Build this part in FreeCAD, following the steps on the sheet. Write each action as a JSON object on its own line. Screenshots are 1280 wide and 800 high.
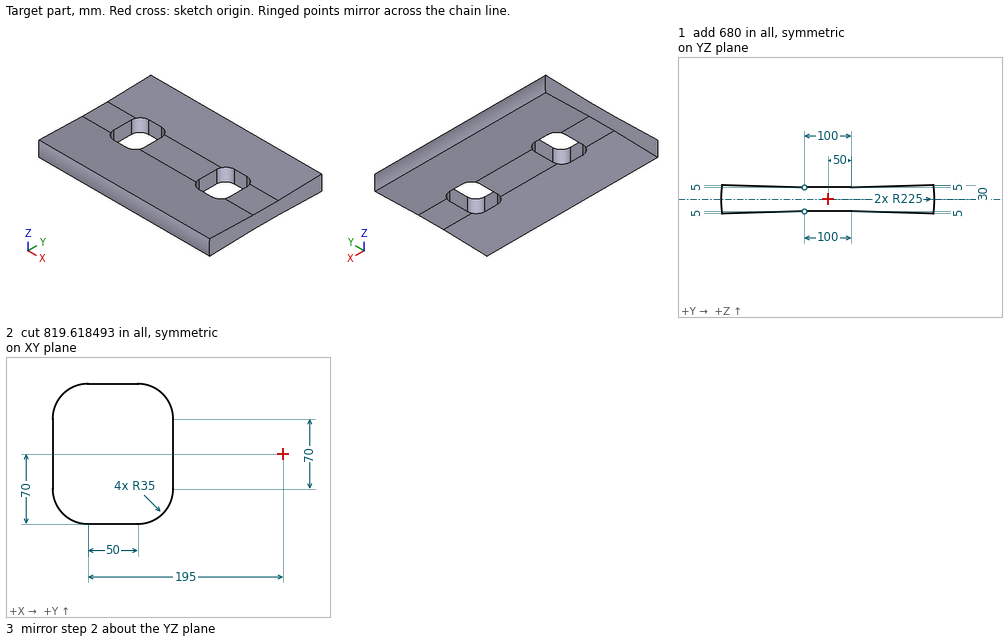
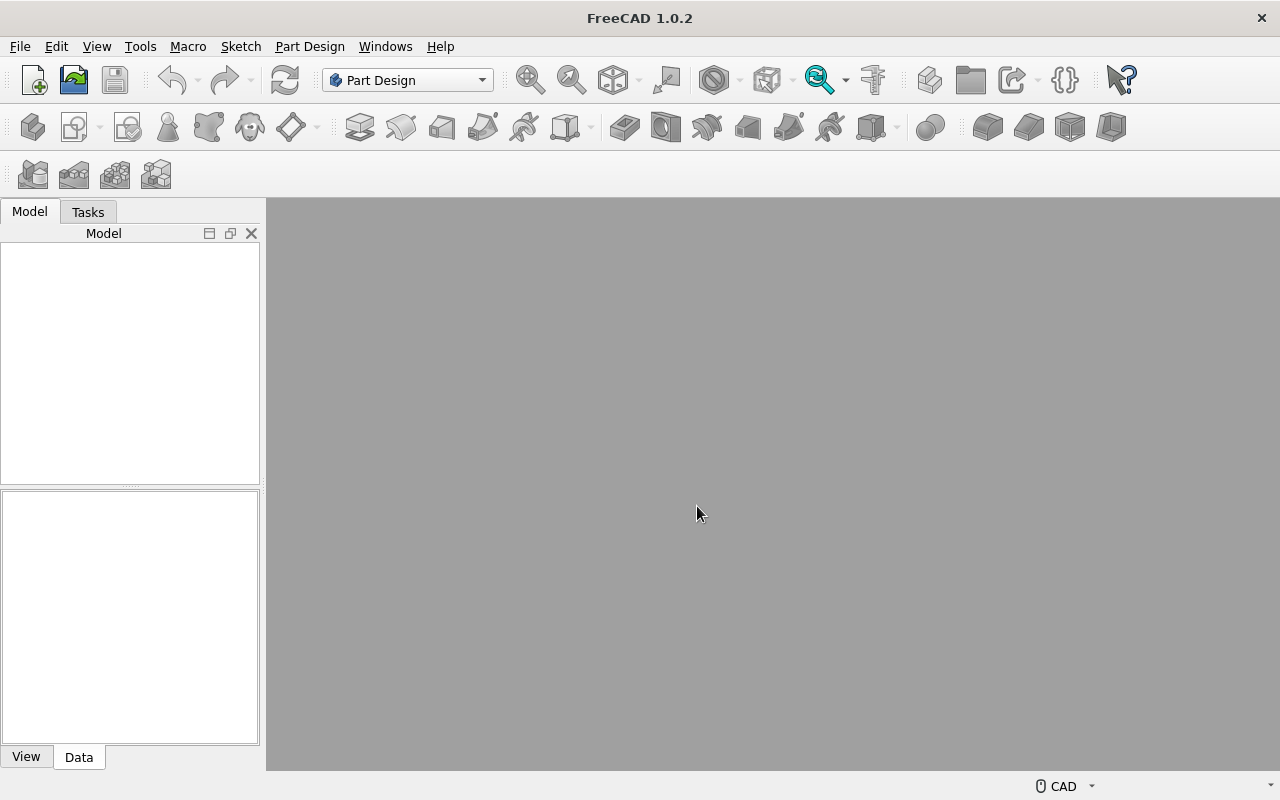
{"action": "key", "text": "ctrl+n"}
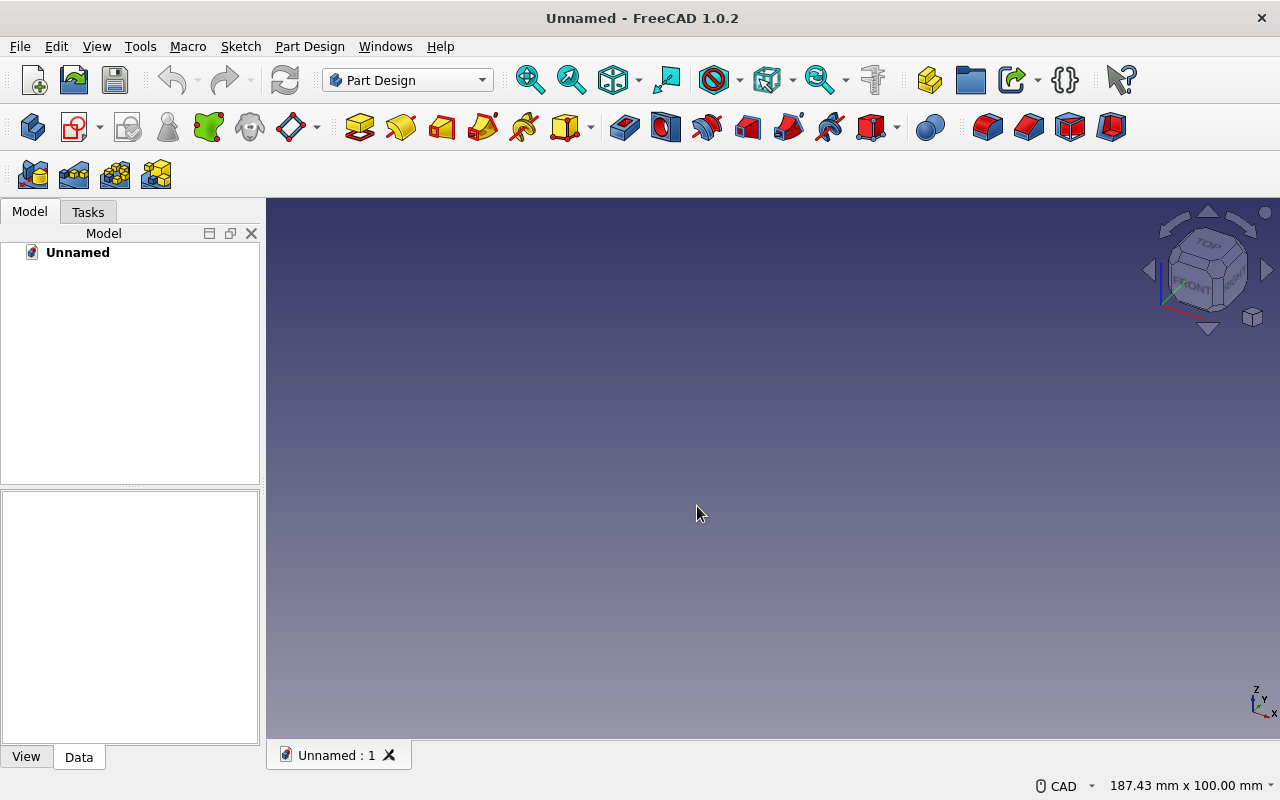
{"action": "left_click", "coordinate": [74, 128]}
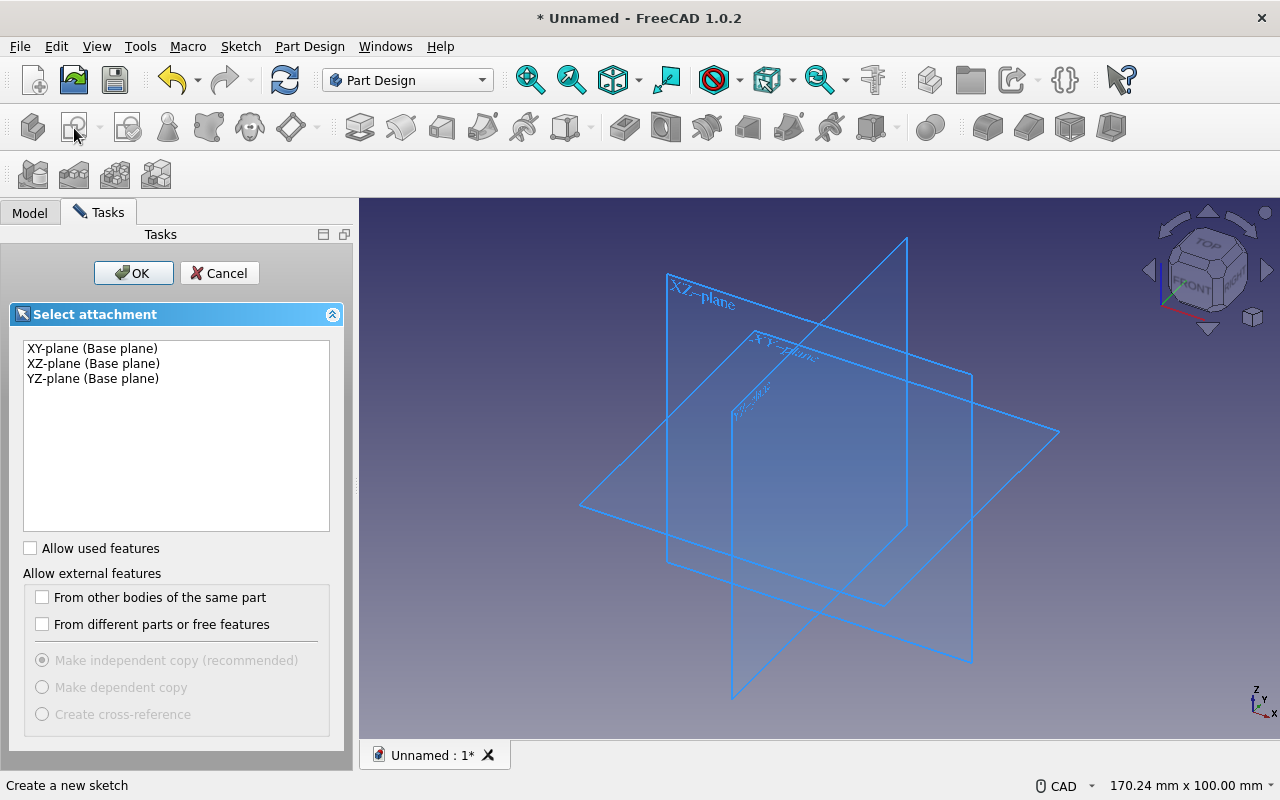
{"action": "left_click", "coordinate": [84, 378]}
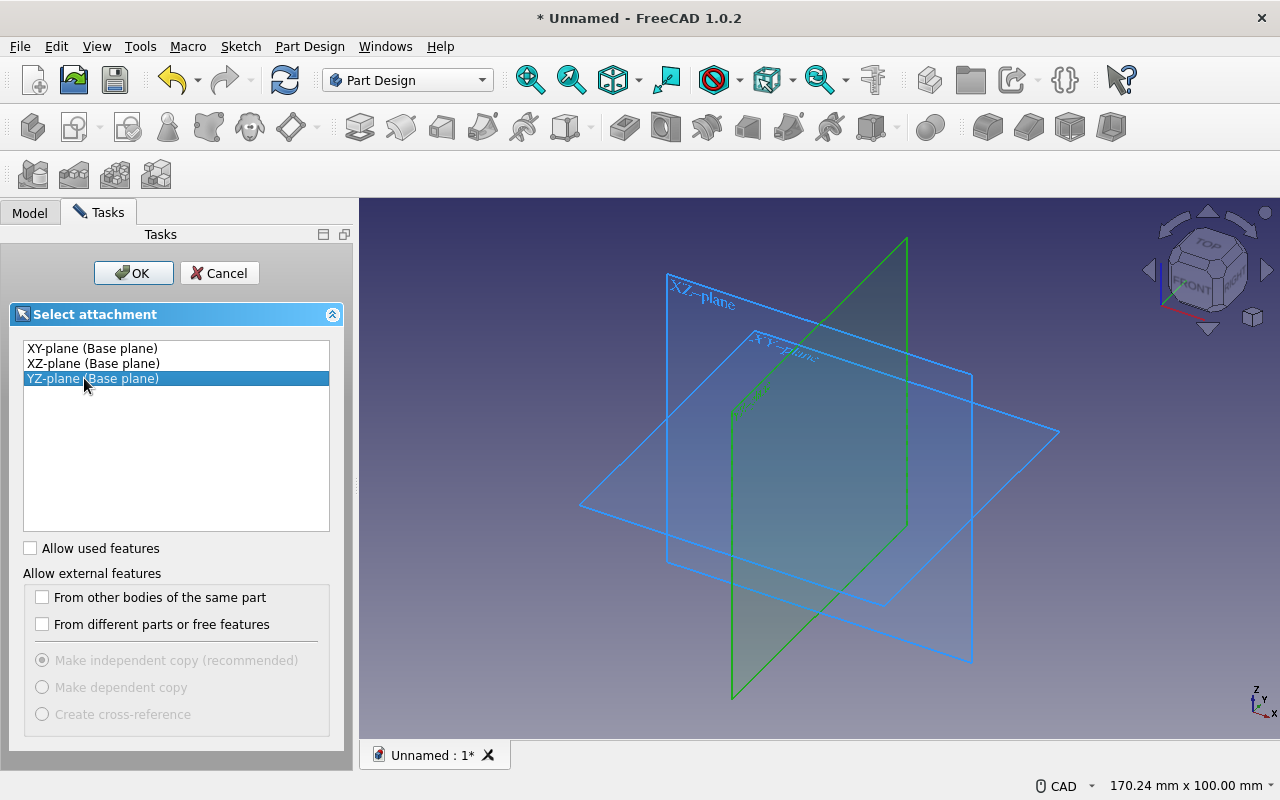
{"action": "left_click", "coordinate": [134, 273]}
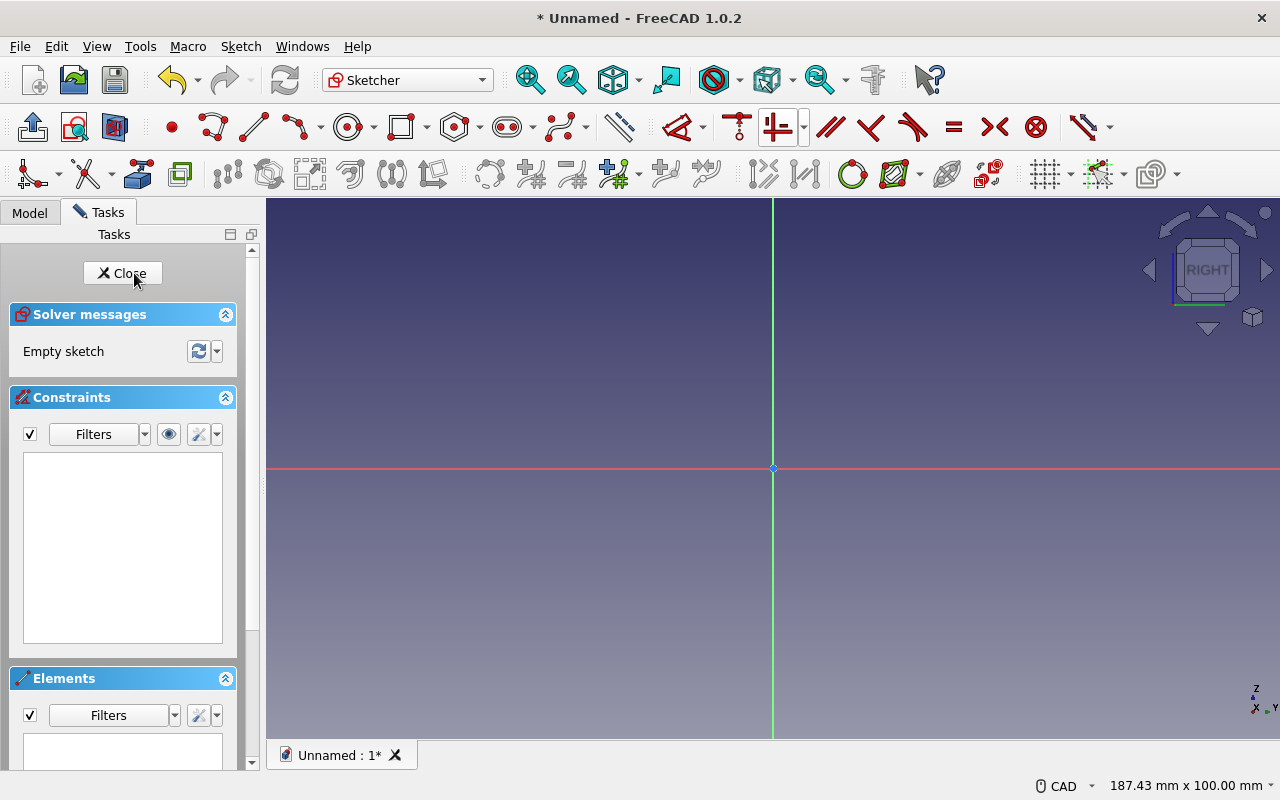
{"action": "scroll", "coordinate": [682, 469], "scroll_direction": "down", "scroll_amount": 7}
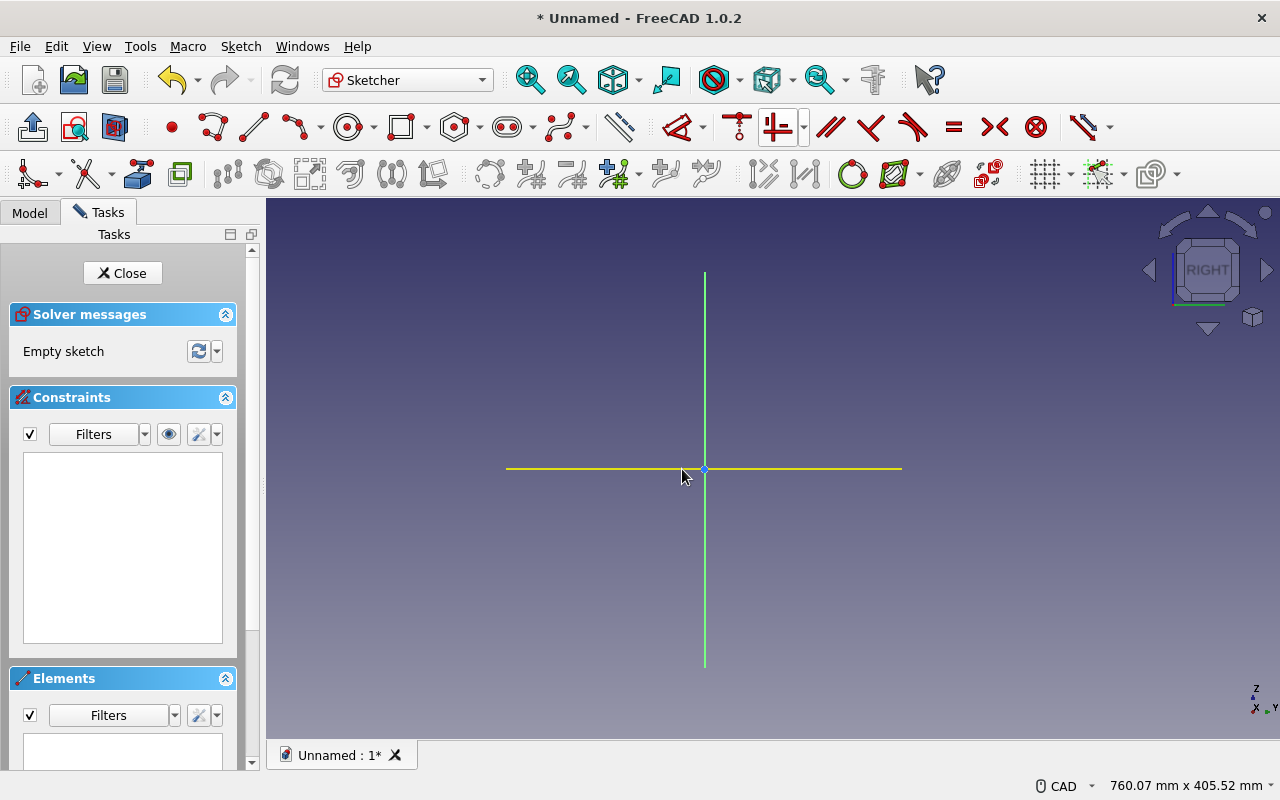
{"action": "key", "text": "g m"}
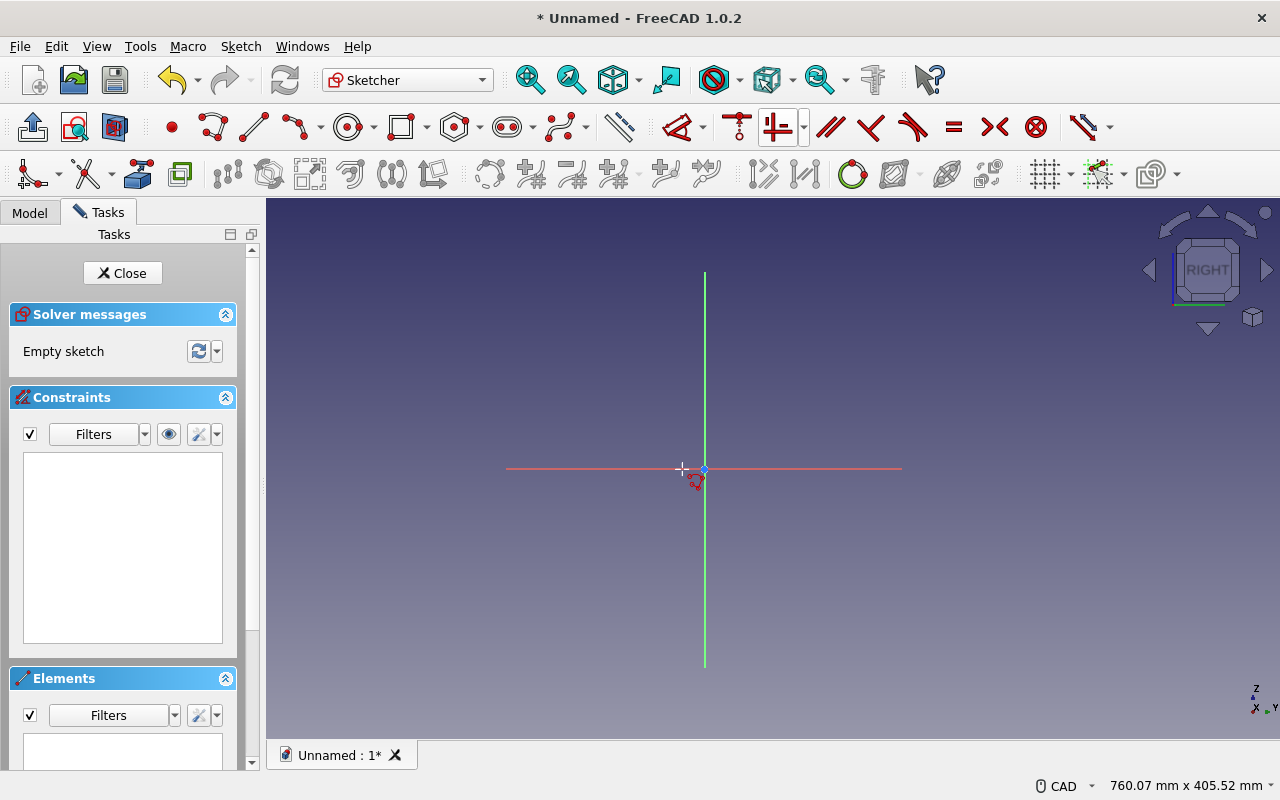
{"action": "left_click", "coordinate": [1002, 429]}
{"action": "left_click", "coordinate": [771, 441]}
{"action": "left_click", "coordinate": [638, 441]}
{"action": "left_click", "coordinate": [407, 429]}
{"action": "right_click", "coordinate": [407, 429]}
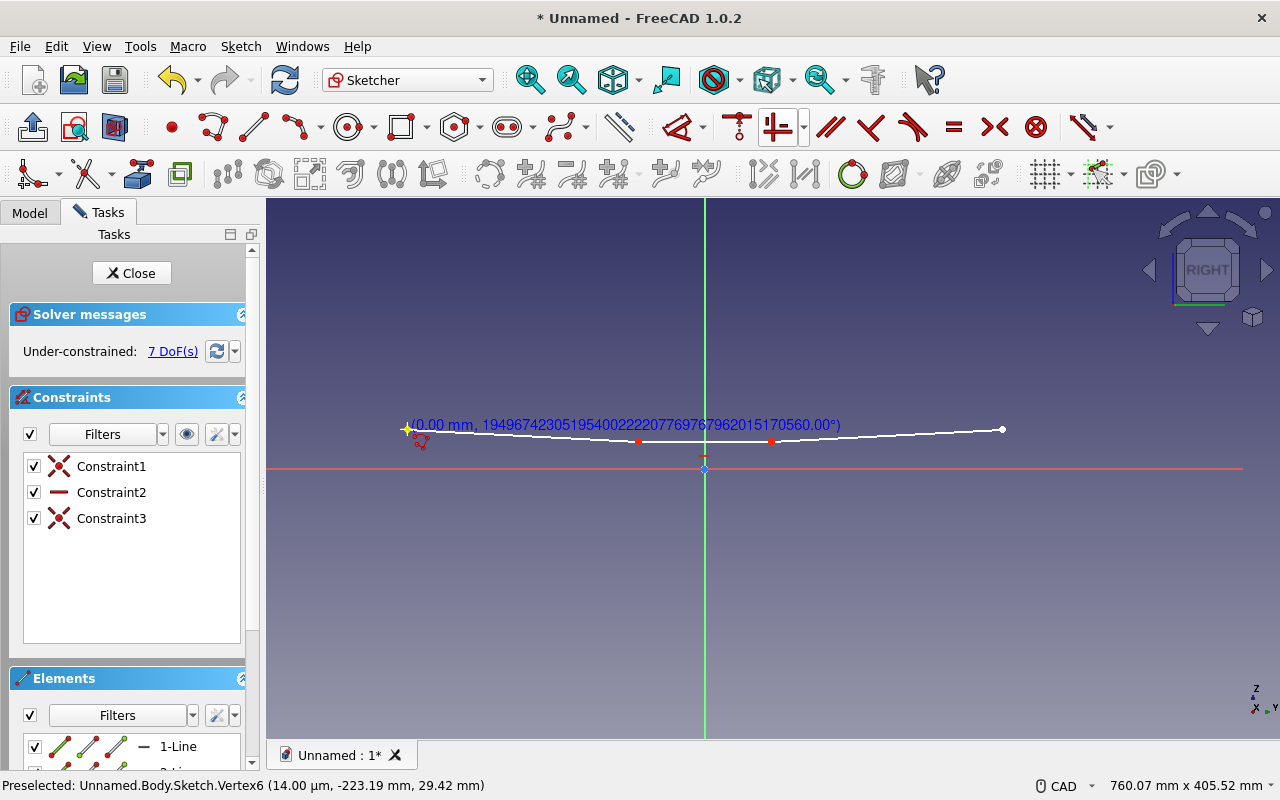
{"action": "left_click", "coordinate": [407, 509]}
{"action": "left_click", "coordinate": [638, 497]}
{"action": "left_click", "coordinate": [771, 497]}
{"action": "left_click", "coordinate": [1002, 509]}
{"action": "right_click", "coordinate": [1002, 509]}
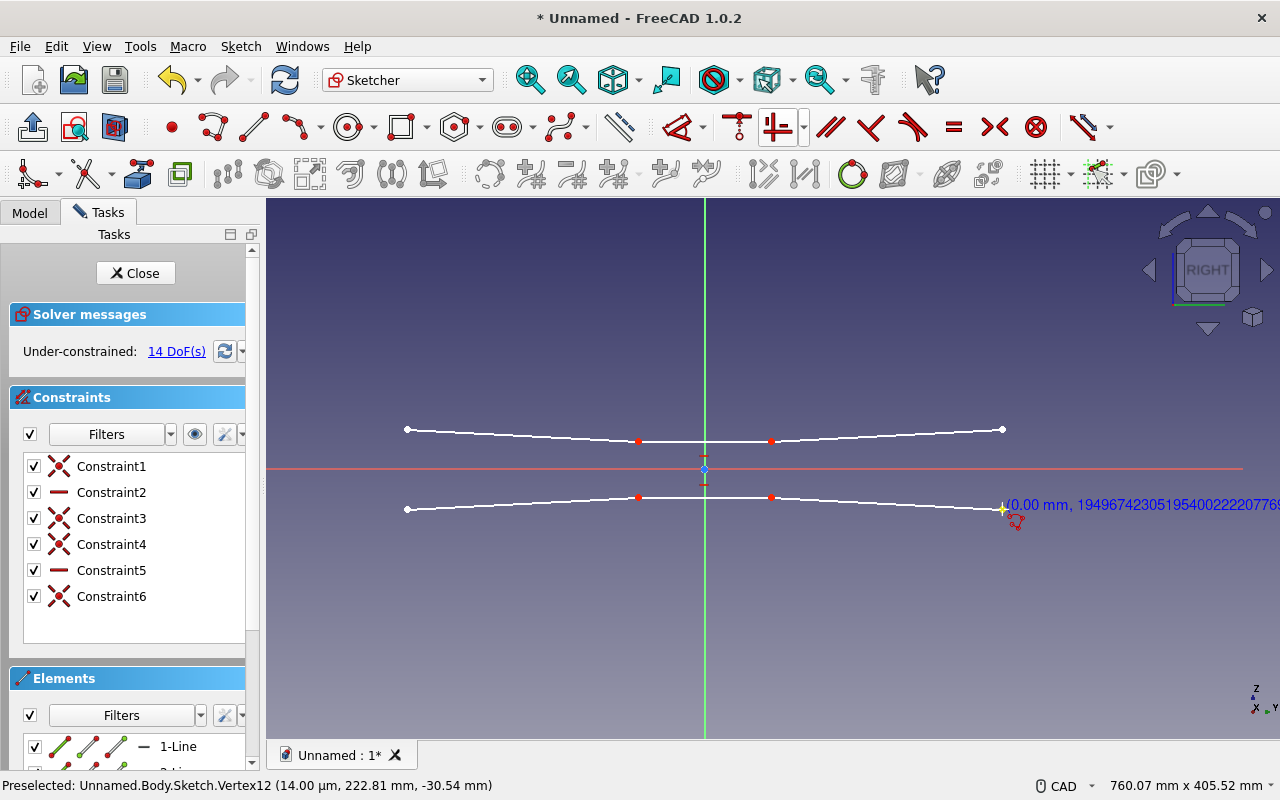
{"action": "key", "text": "g 3 a"}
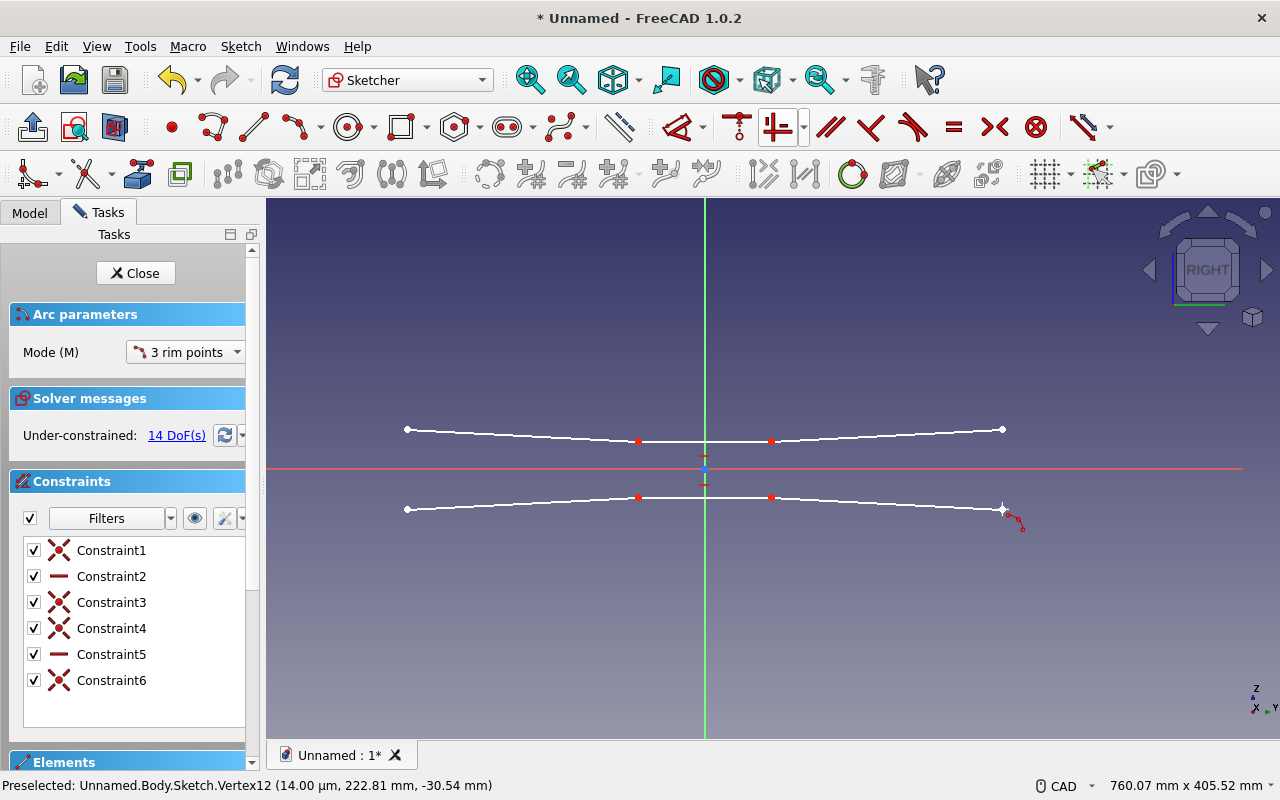
{"action": "left_click", "coordinate": [407, 430]}
{"action": "left_click", "coordinate": [407, 510]}